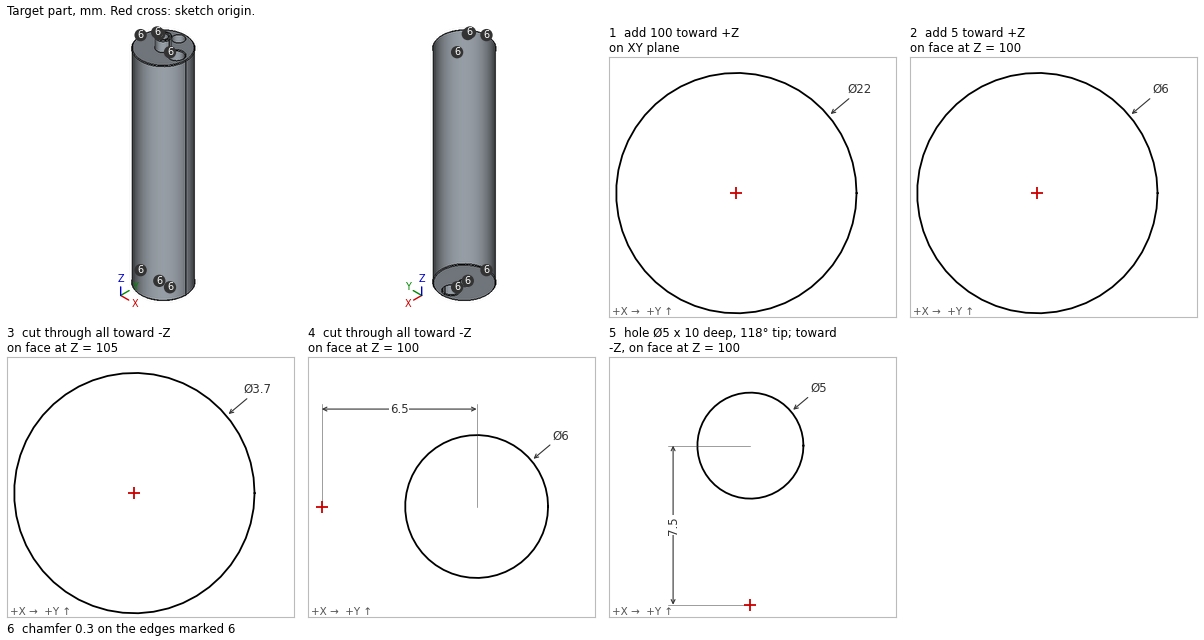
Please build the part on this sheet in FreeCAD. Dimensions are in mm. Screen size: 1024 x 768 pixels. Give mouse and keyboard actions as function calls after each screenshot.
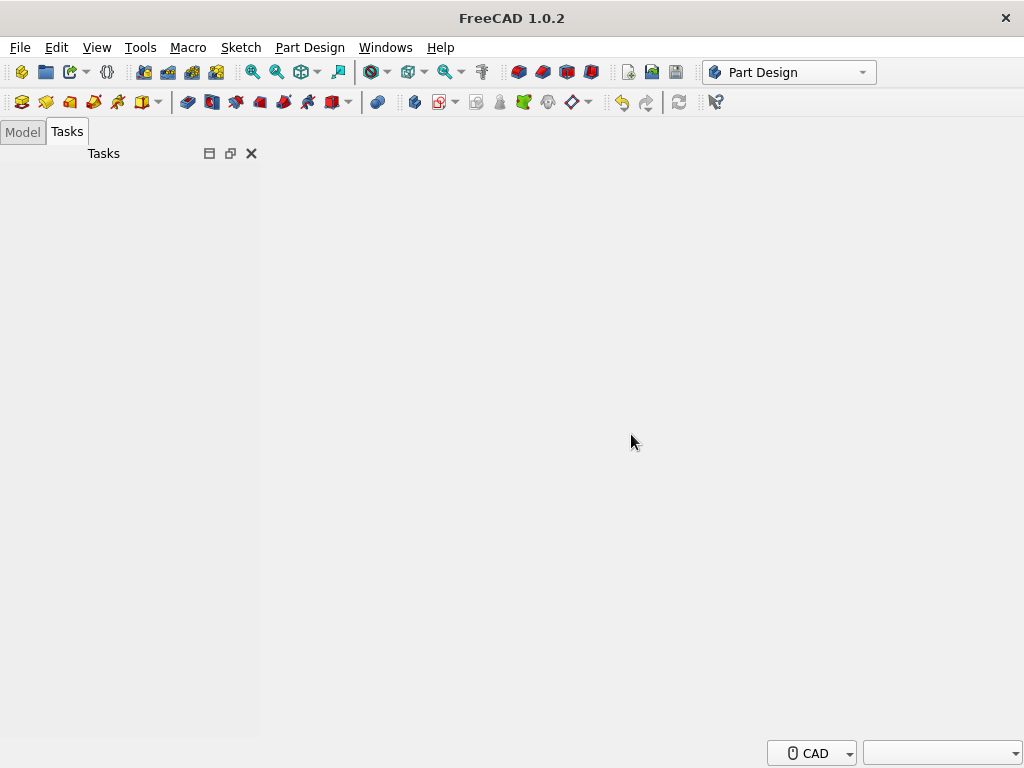
click(628, 72)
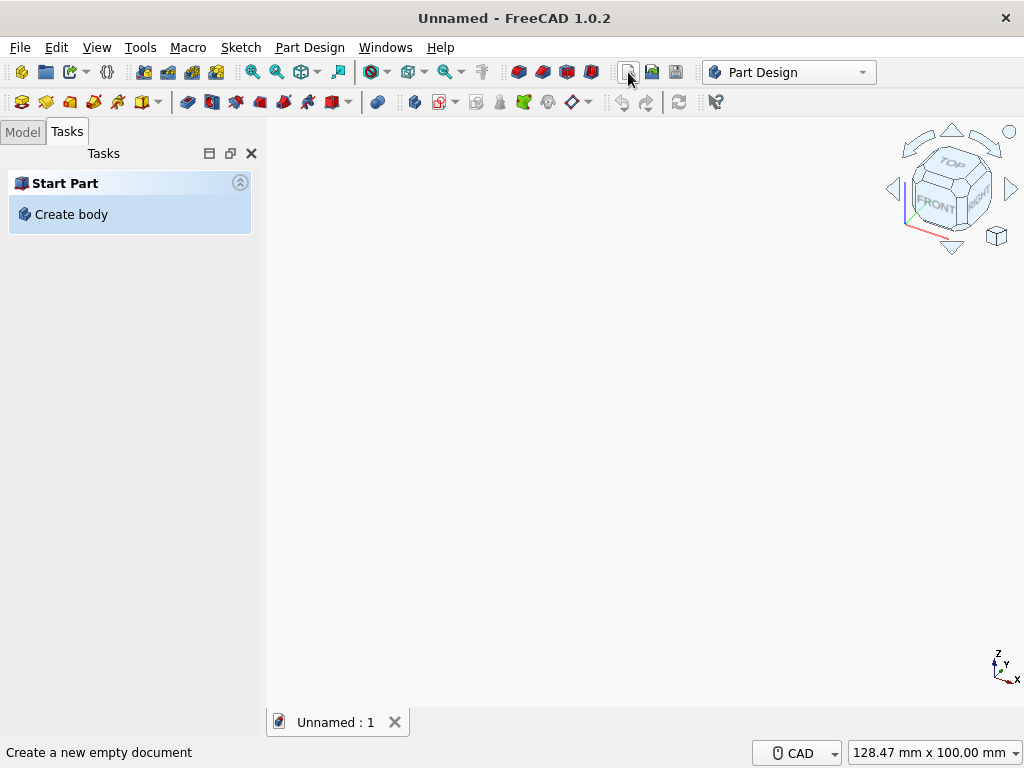
click(440, 102)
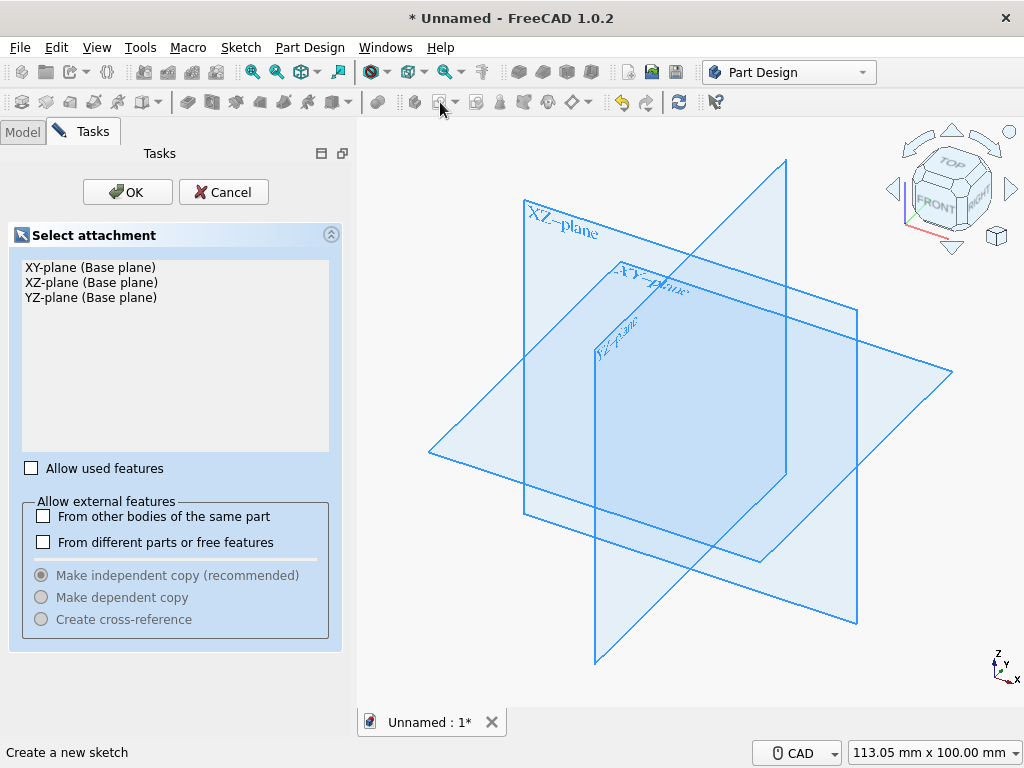
click(82, 268)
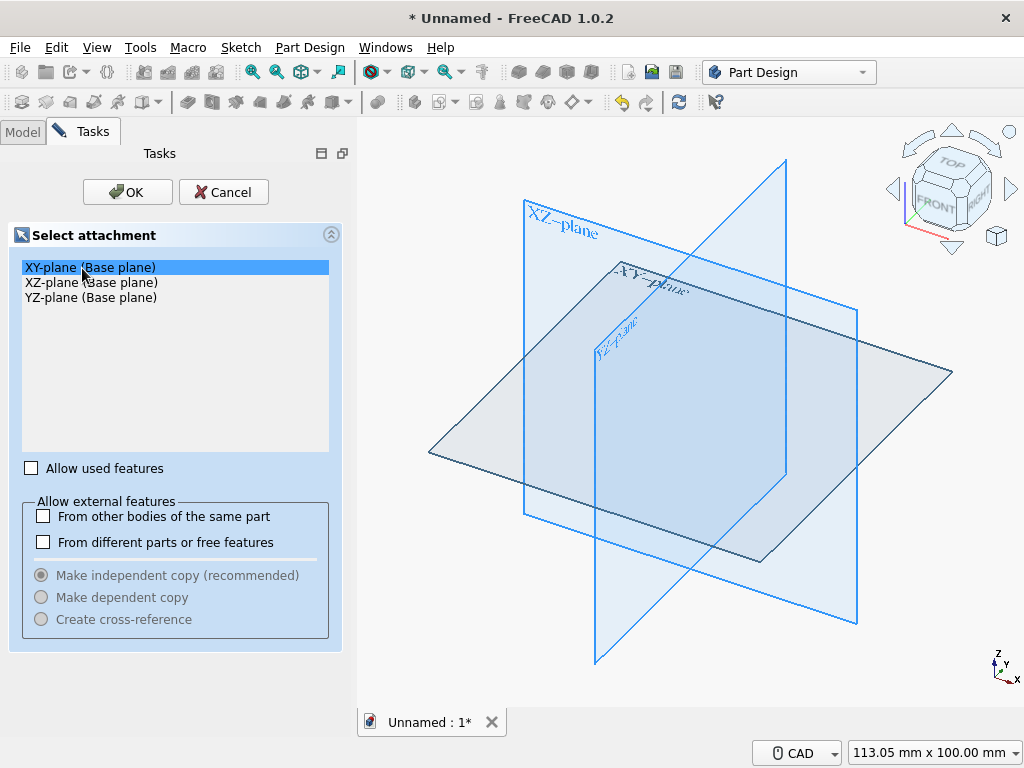
click(128, 192)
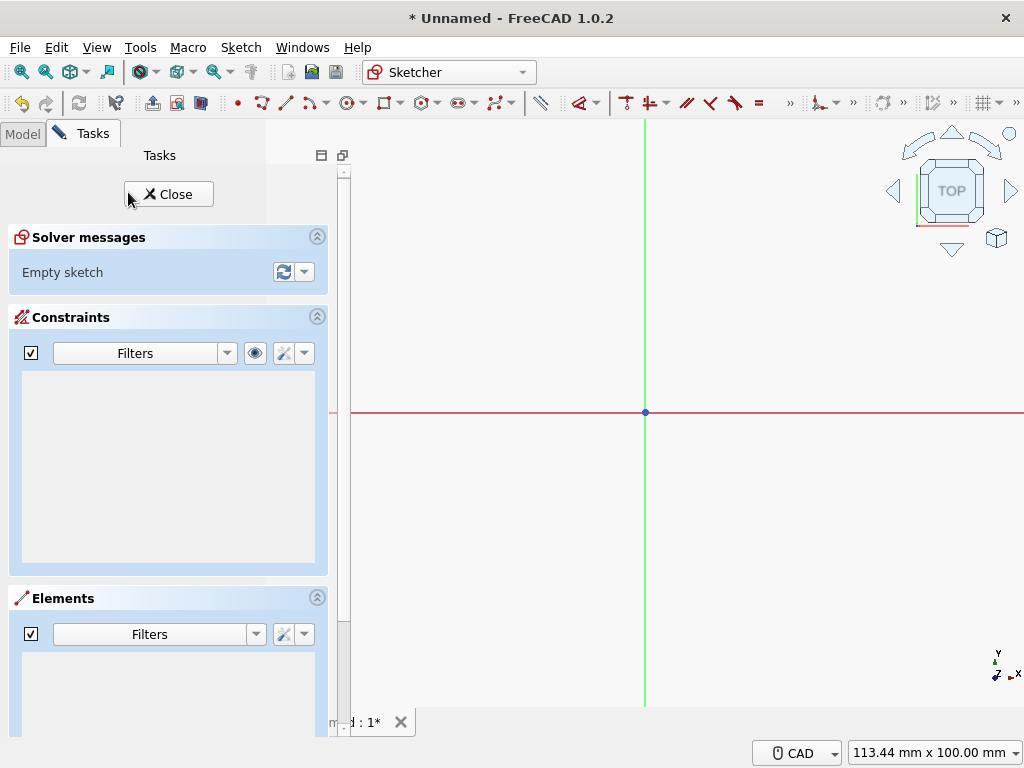
scroll(685, 413, up, 5)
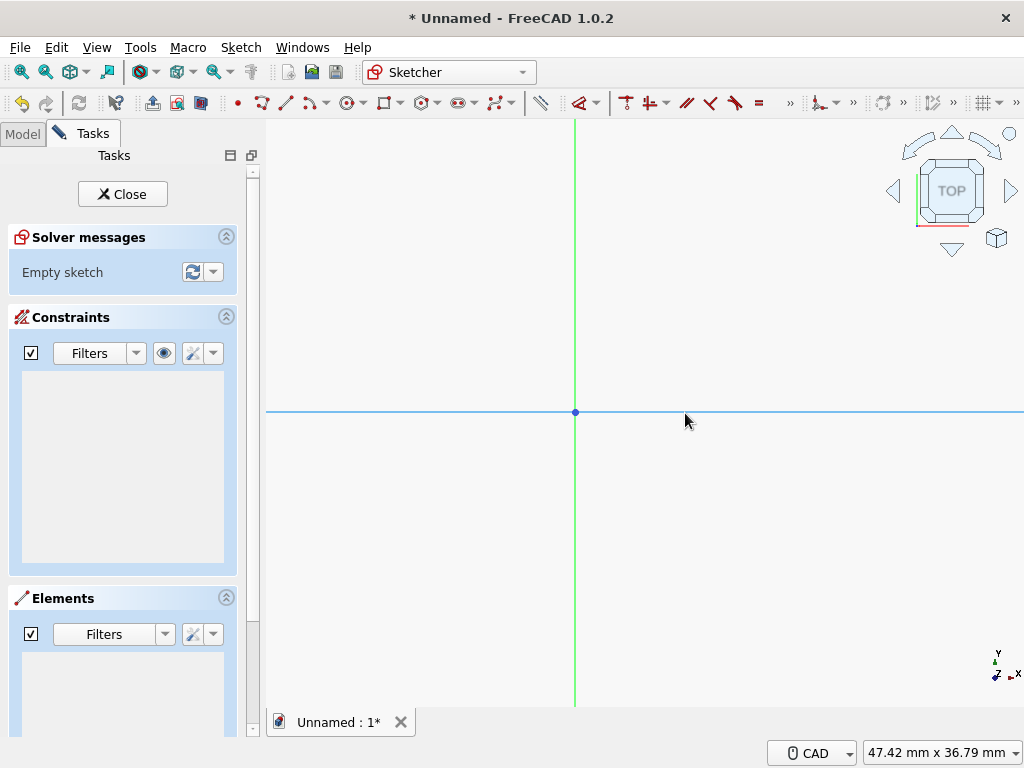
key(g)
key(c)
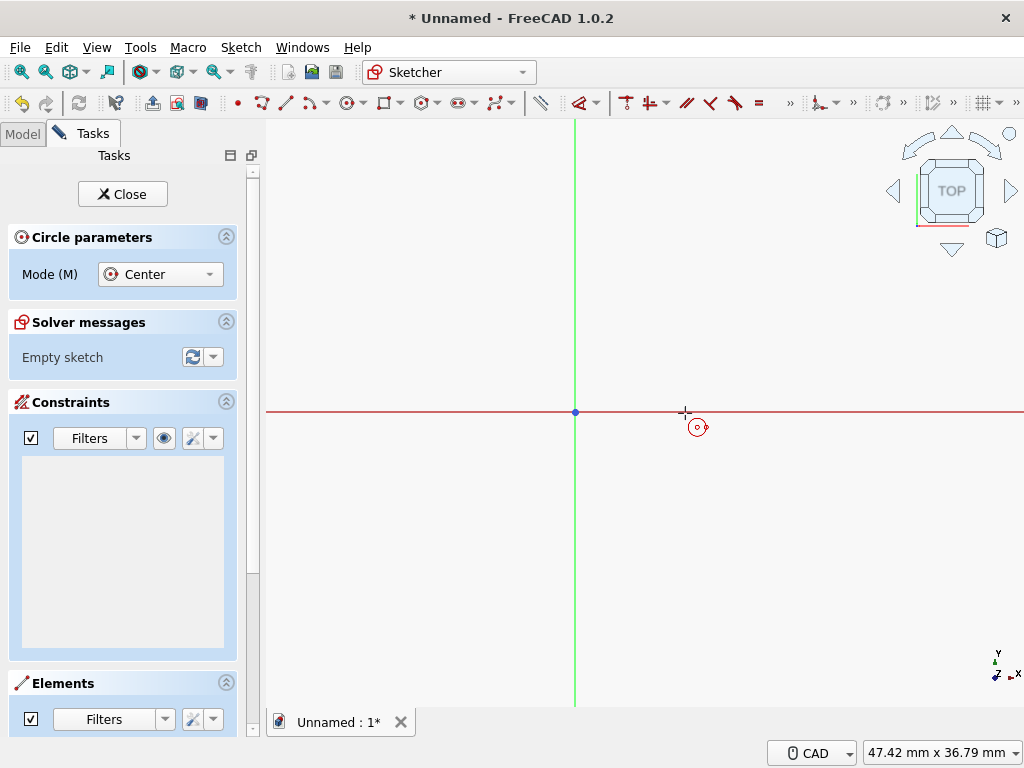
click(575, 412)
click(700, 288)
key(Escape)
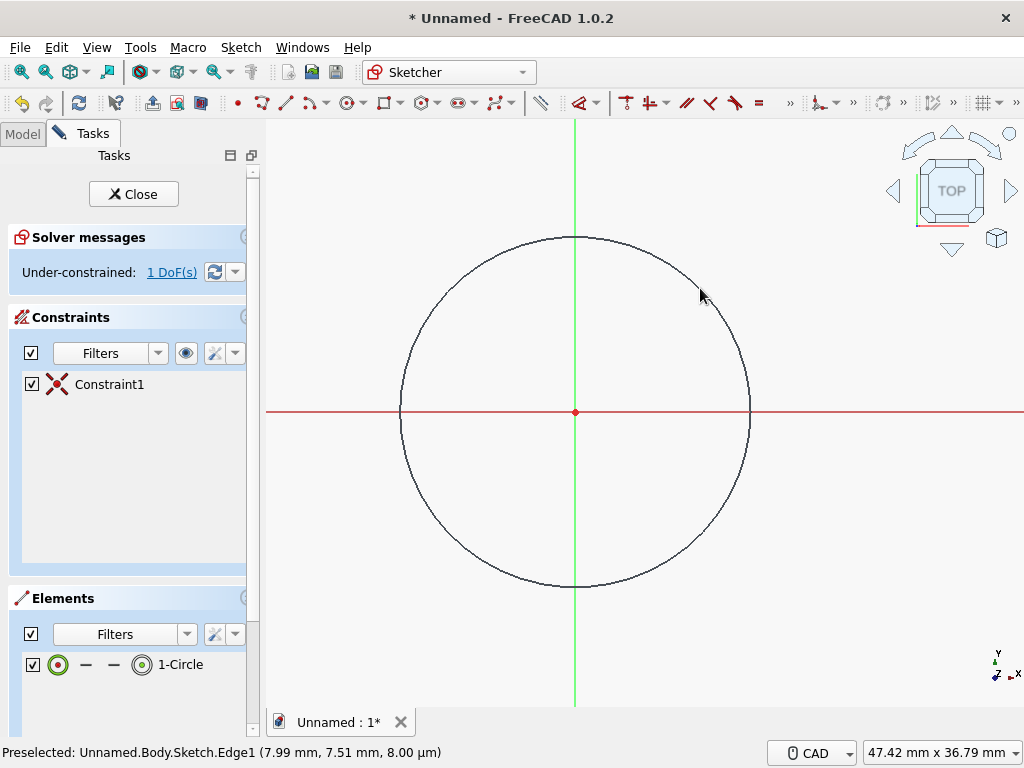
click(699, 288)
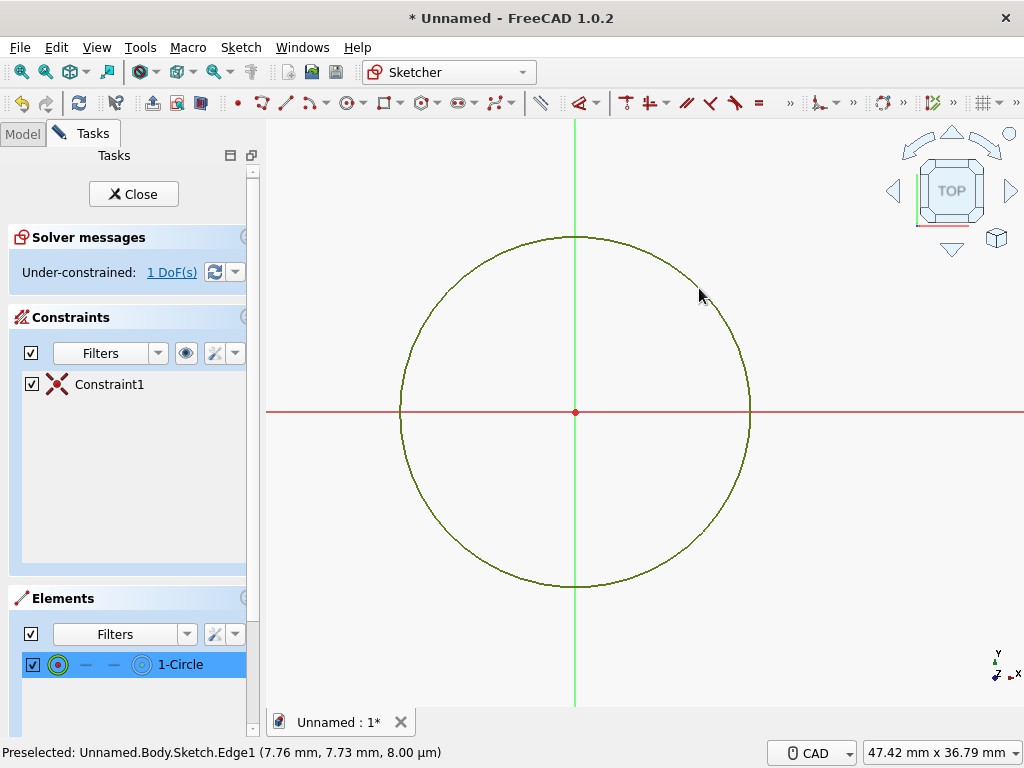
key(k)
key(o)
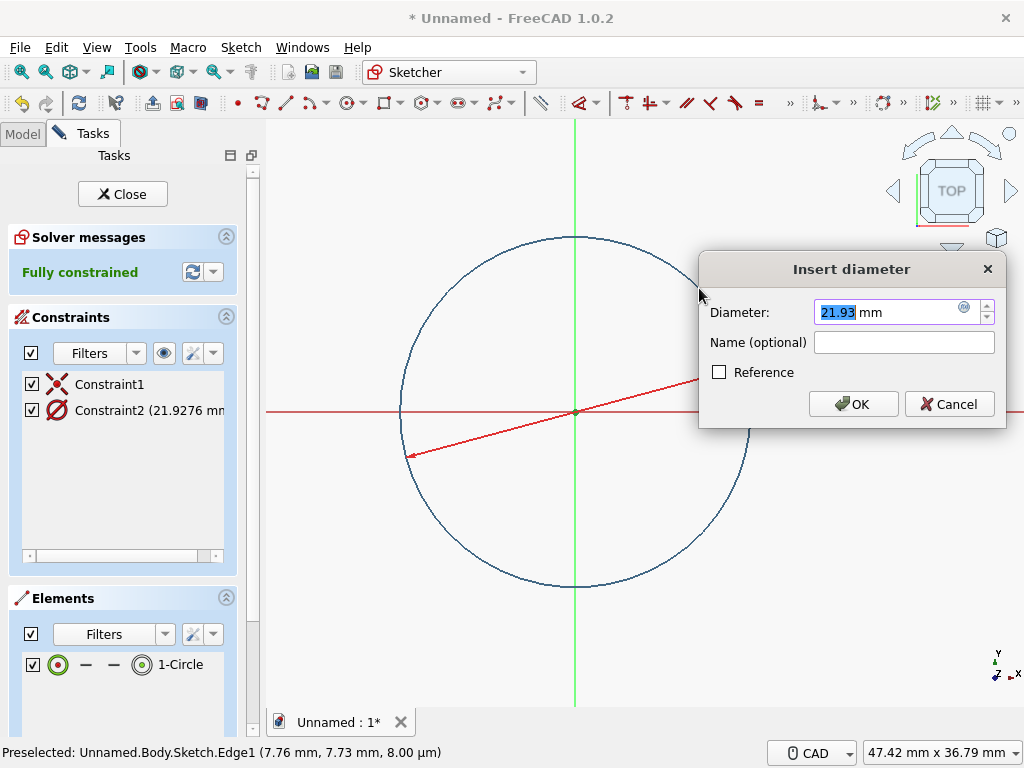
text(22)
key(Return)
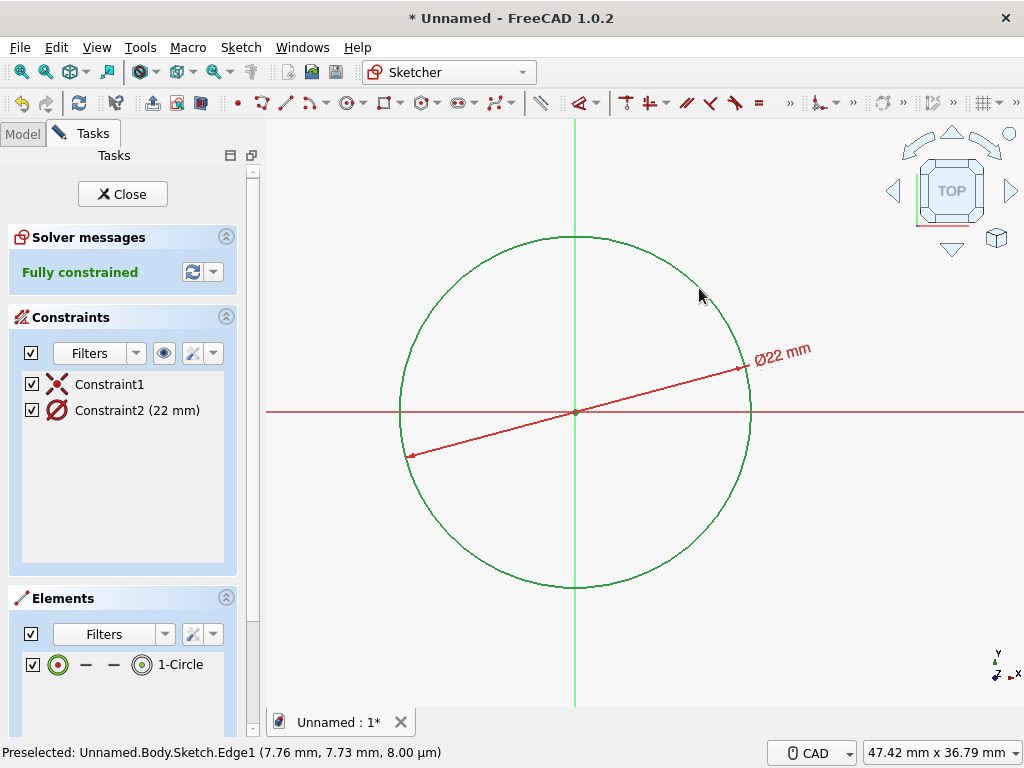
click(123, 194)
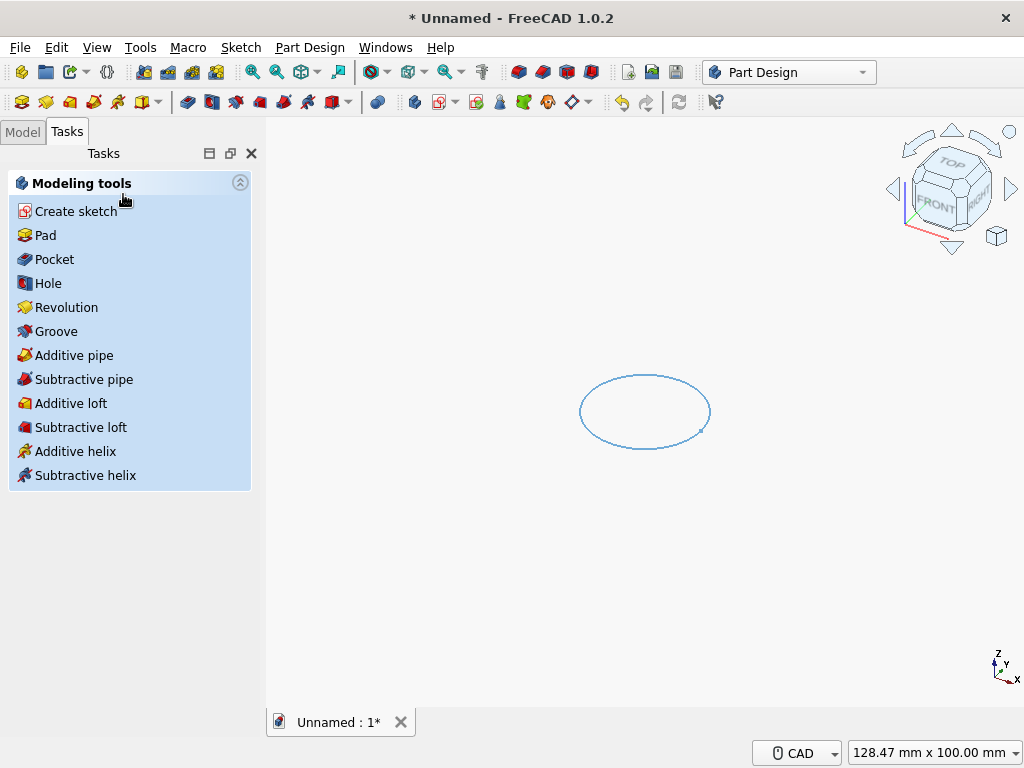
click(22, 102)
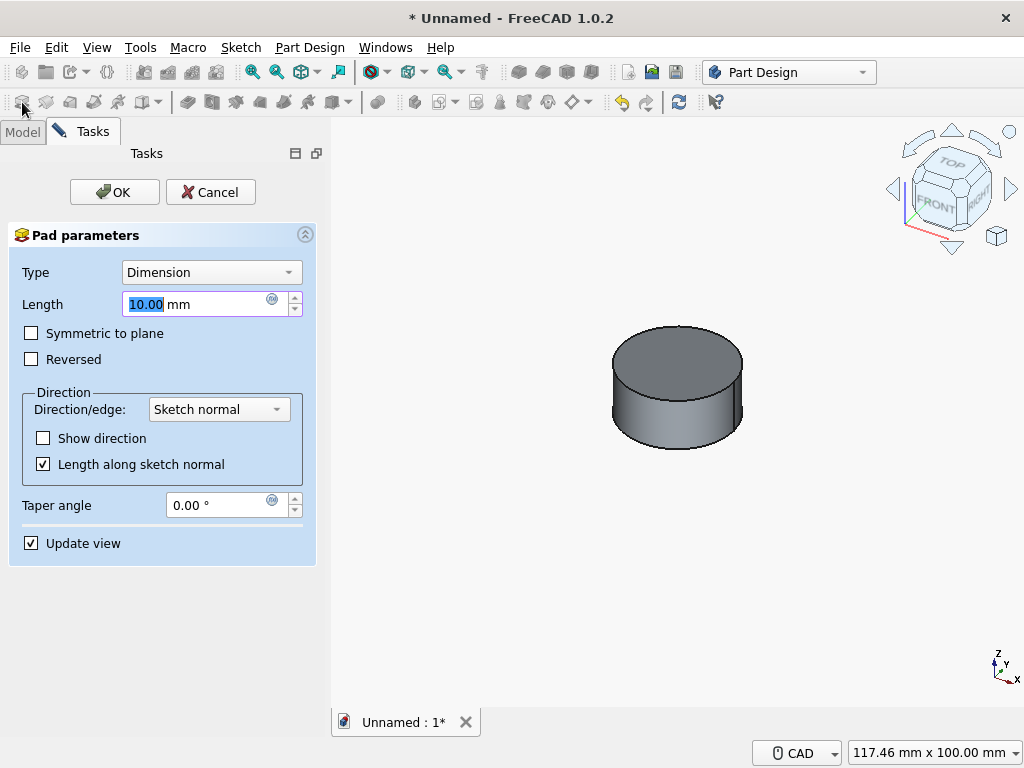
text(100)
key(Tab)